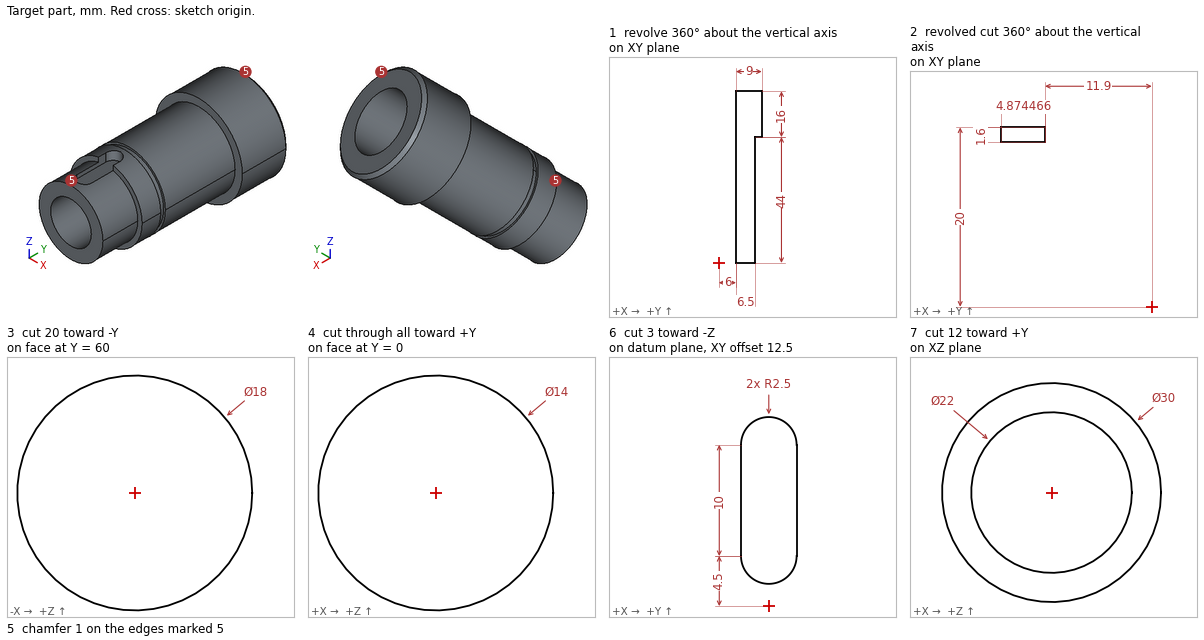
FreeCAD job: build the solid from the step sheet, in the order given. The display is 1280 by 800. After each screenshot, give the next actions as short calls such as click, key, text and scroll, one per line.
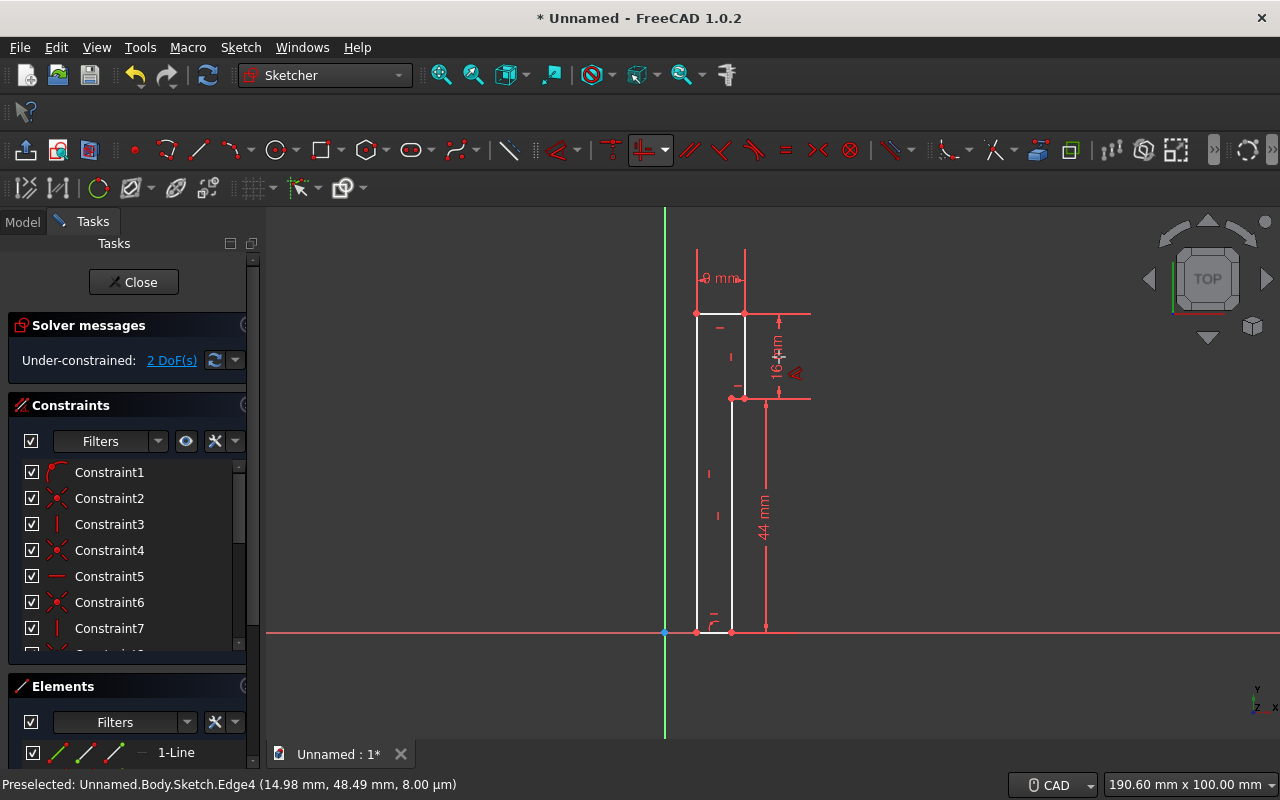
scroll(697, 633, up, 2)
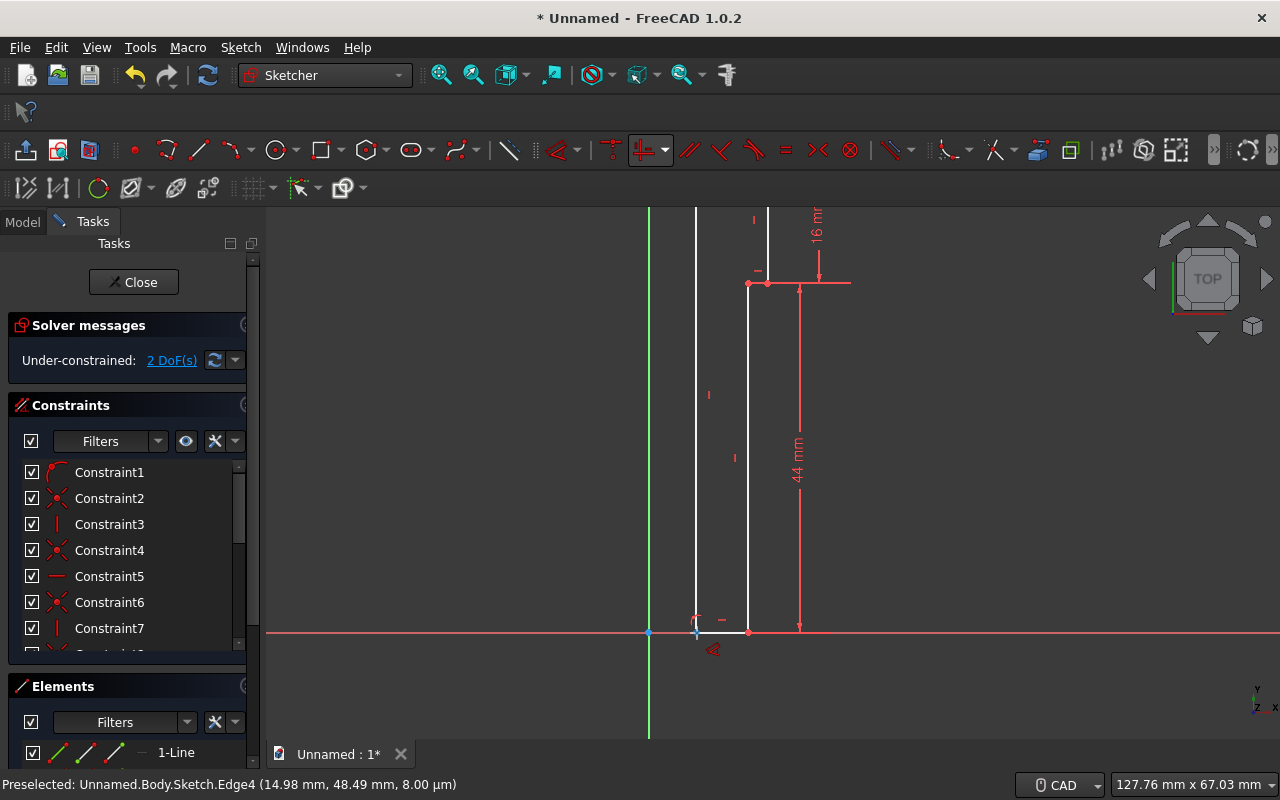
click(696, 633)
click(673, 667)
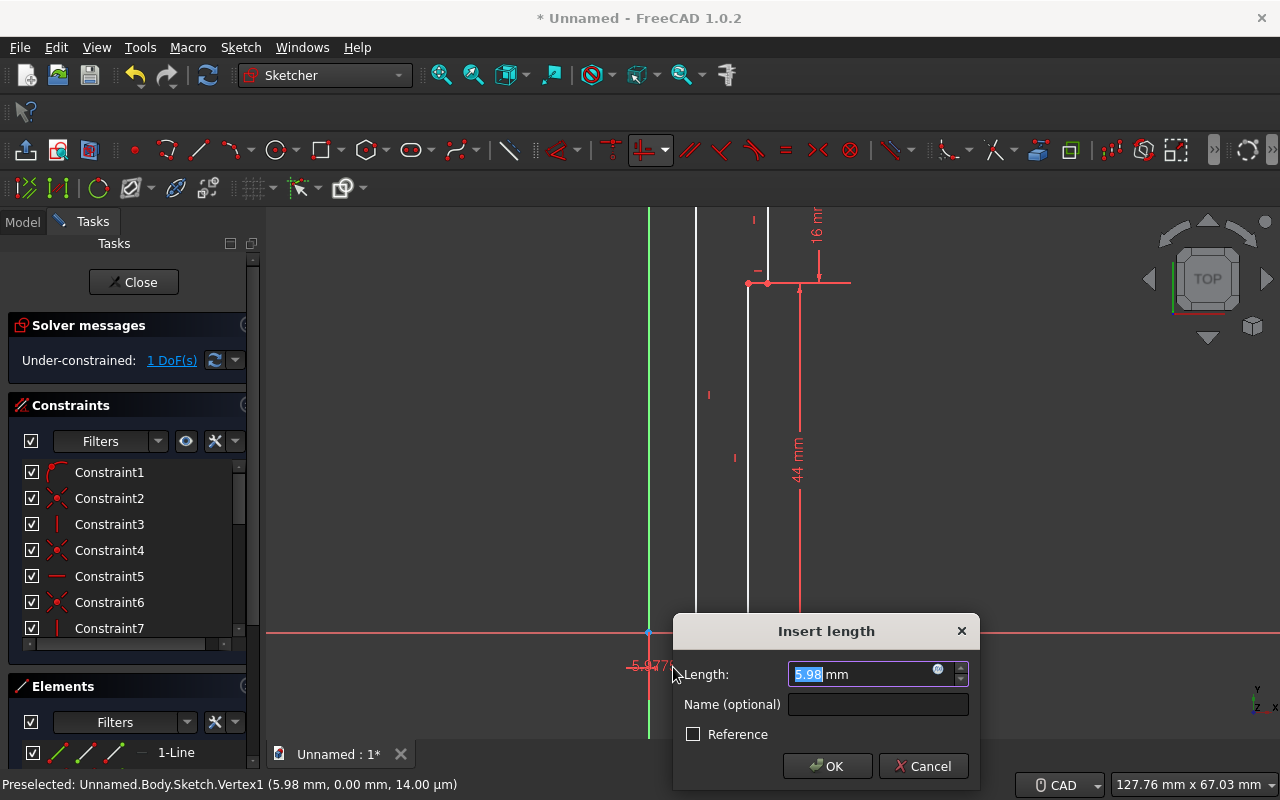
text(6)
key(Return)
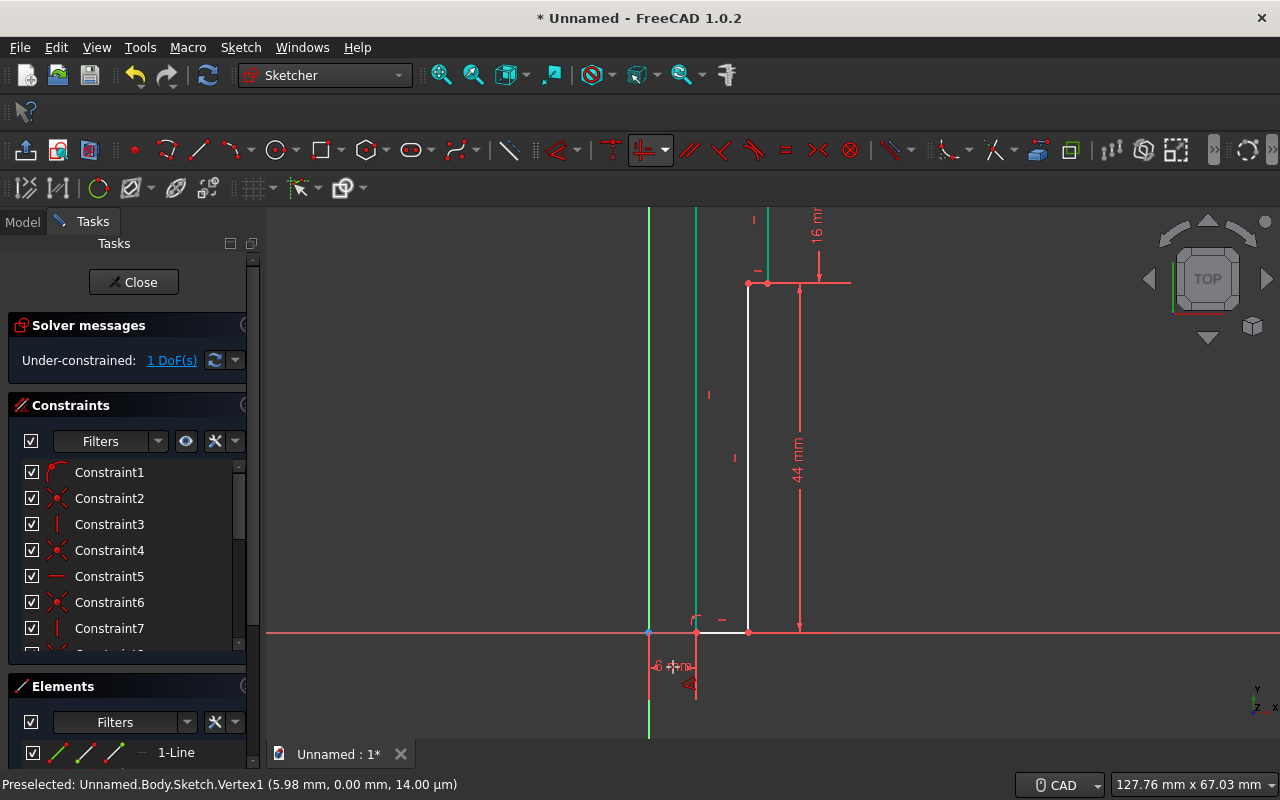
click(712, 633)
click(722, 599)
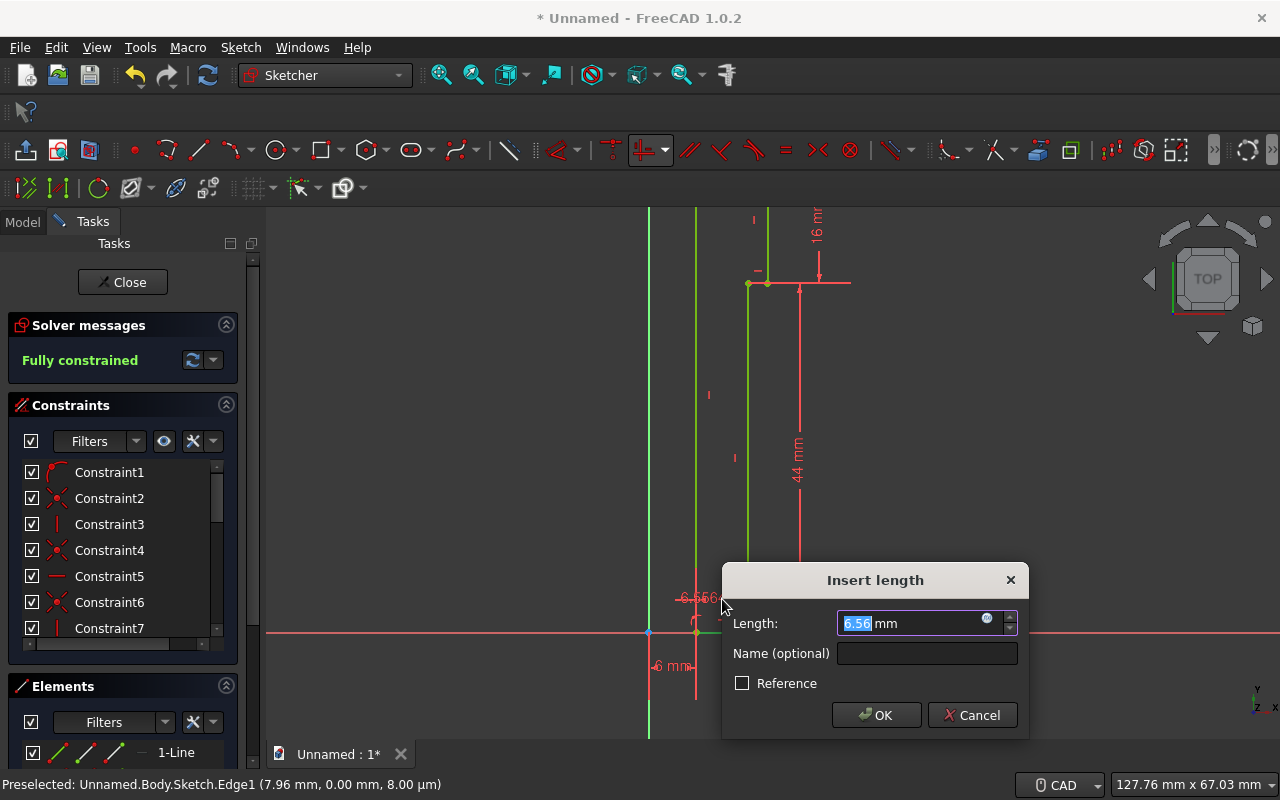
text(6.5)
key(Return)
key(Escape)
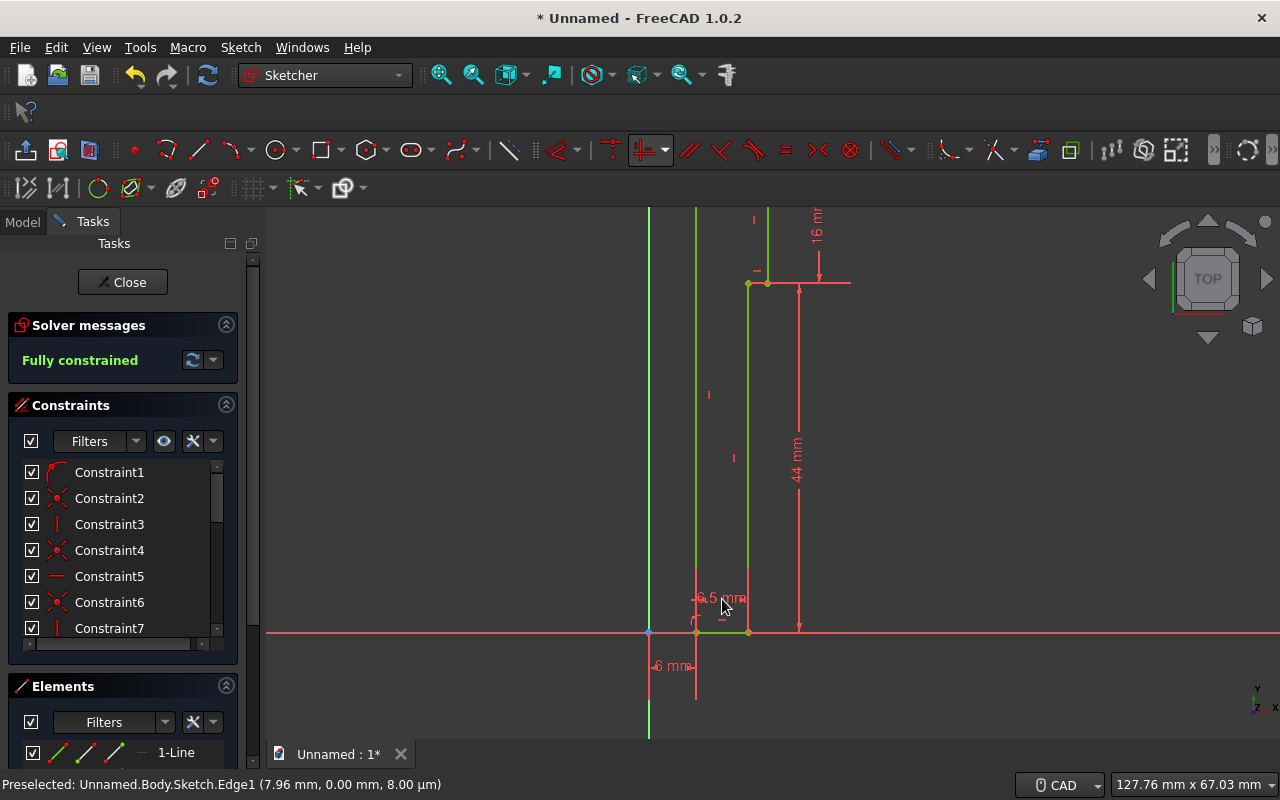
click(123, 282)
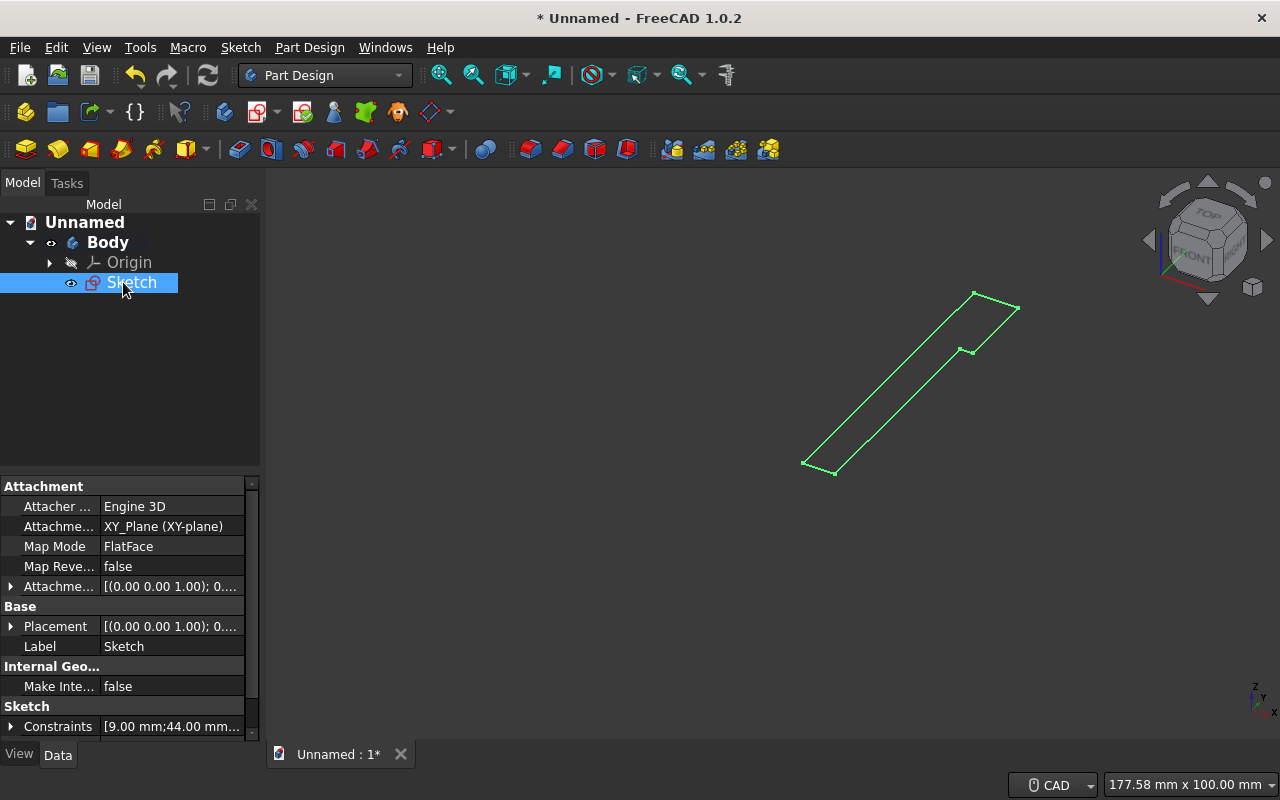
click(58, 150)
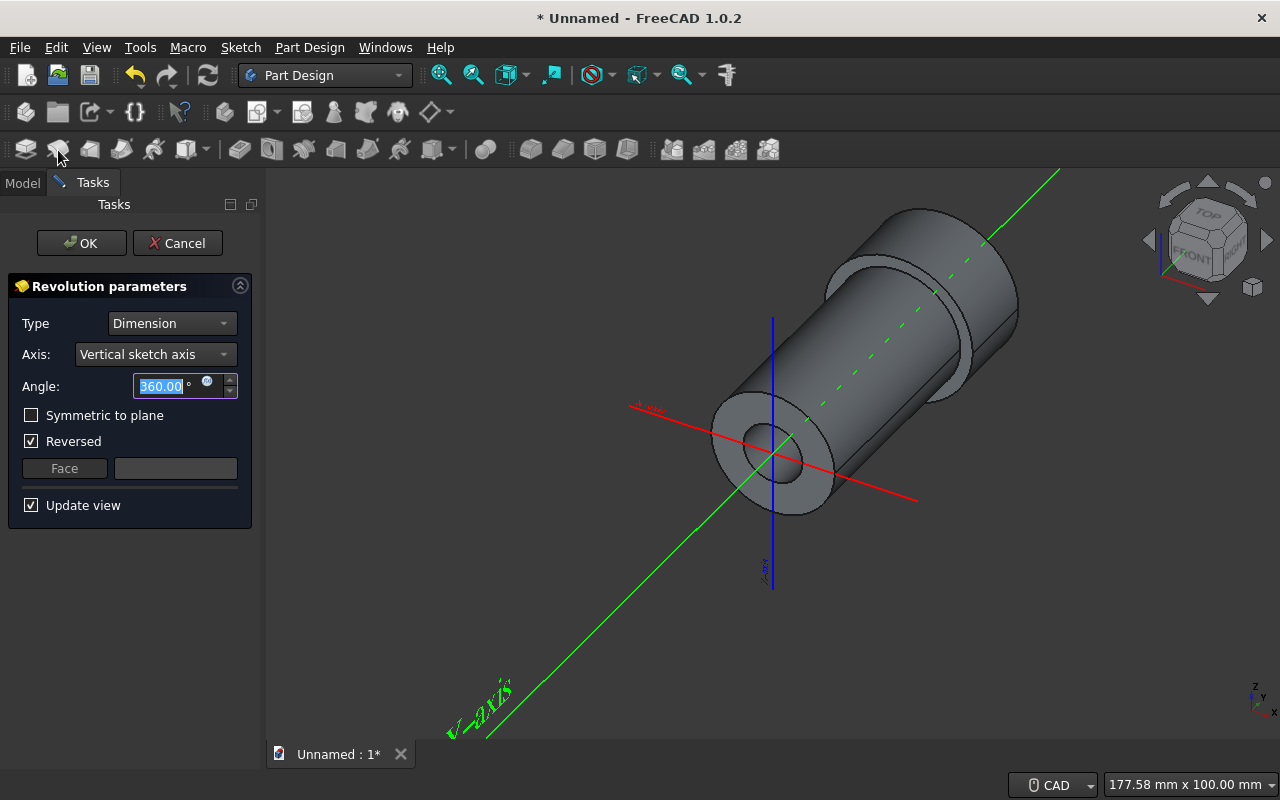
click(82, 243)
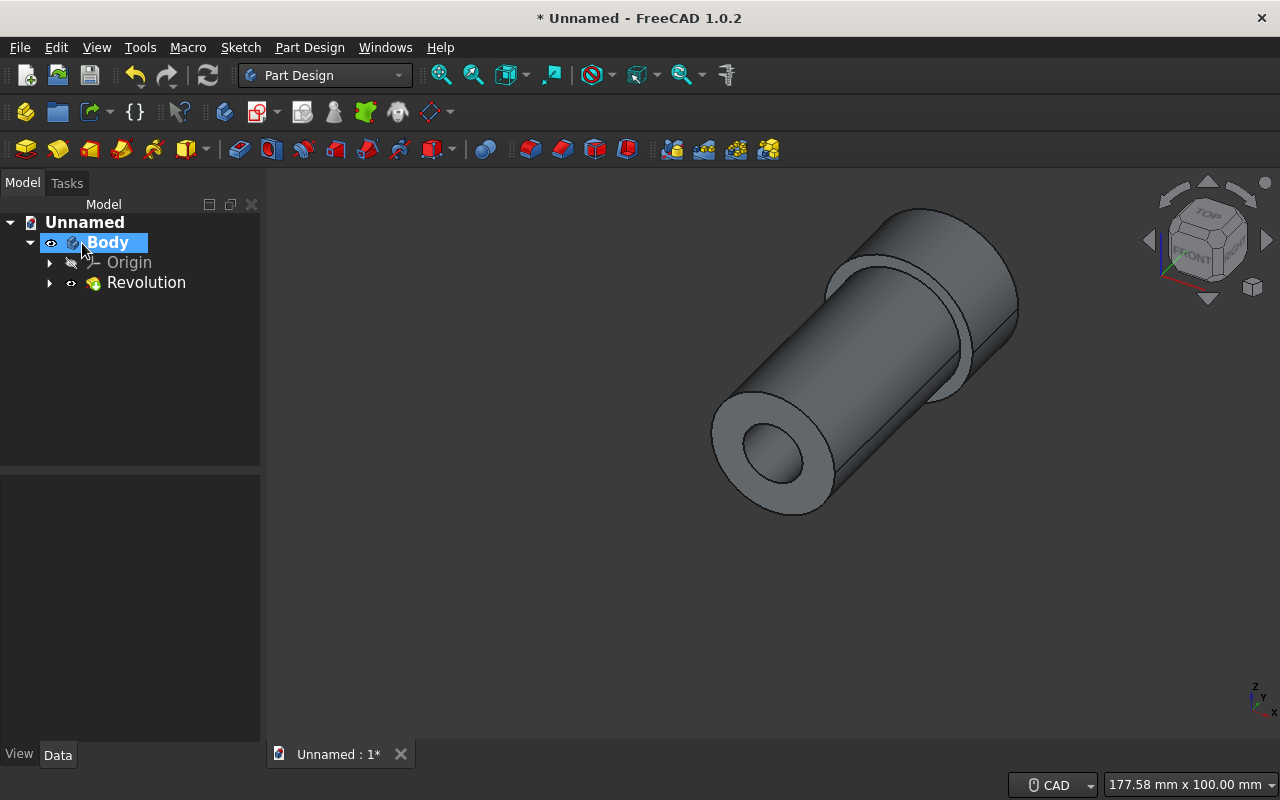
click(258, 112)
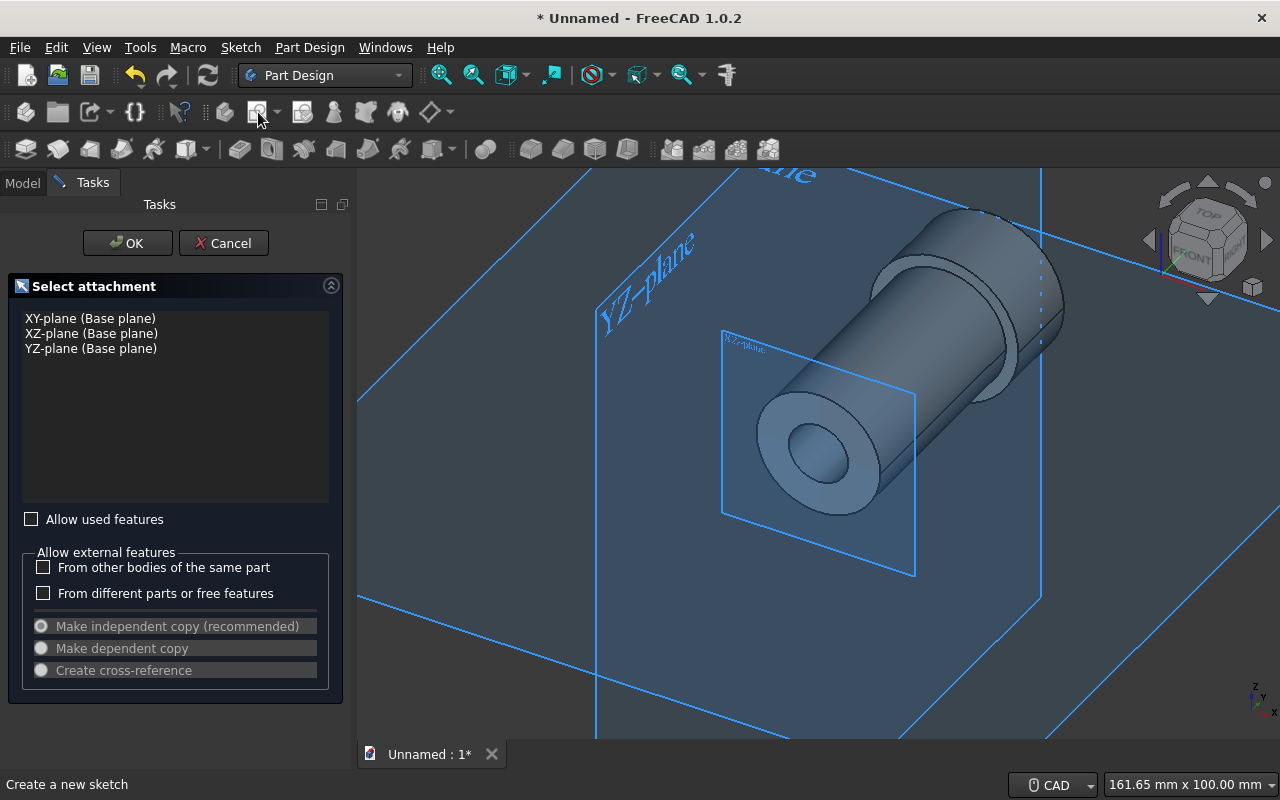
click(82, 318)